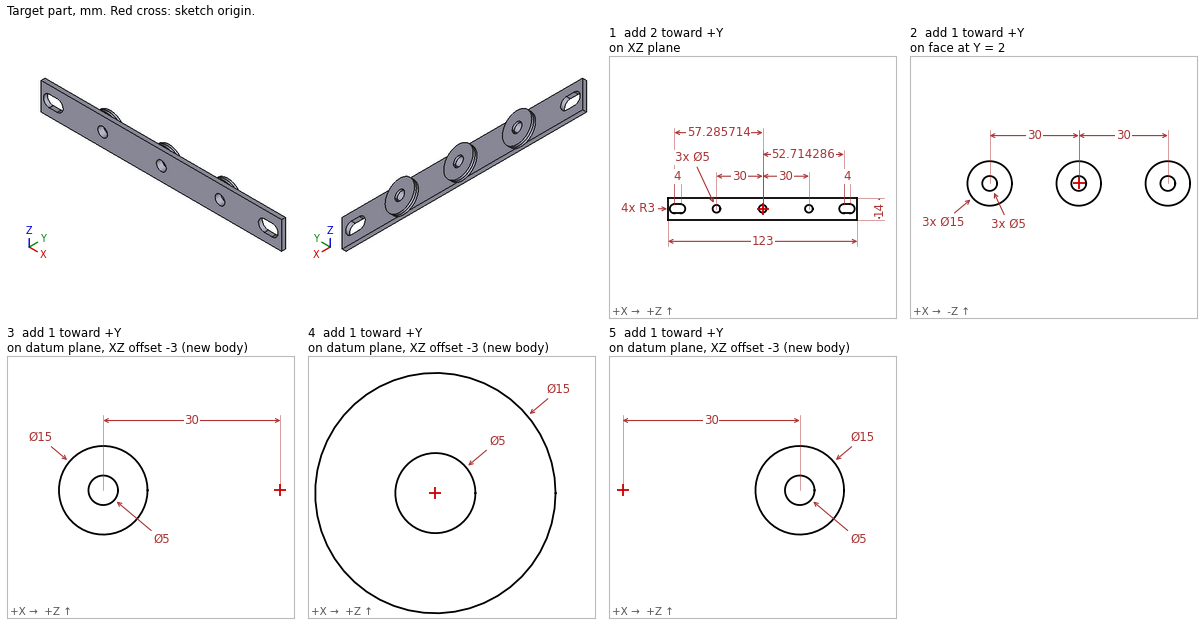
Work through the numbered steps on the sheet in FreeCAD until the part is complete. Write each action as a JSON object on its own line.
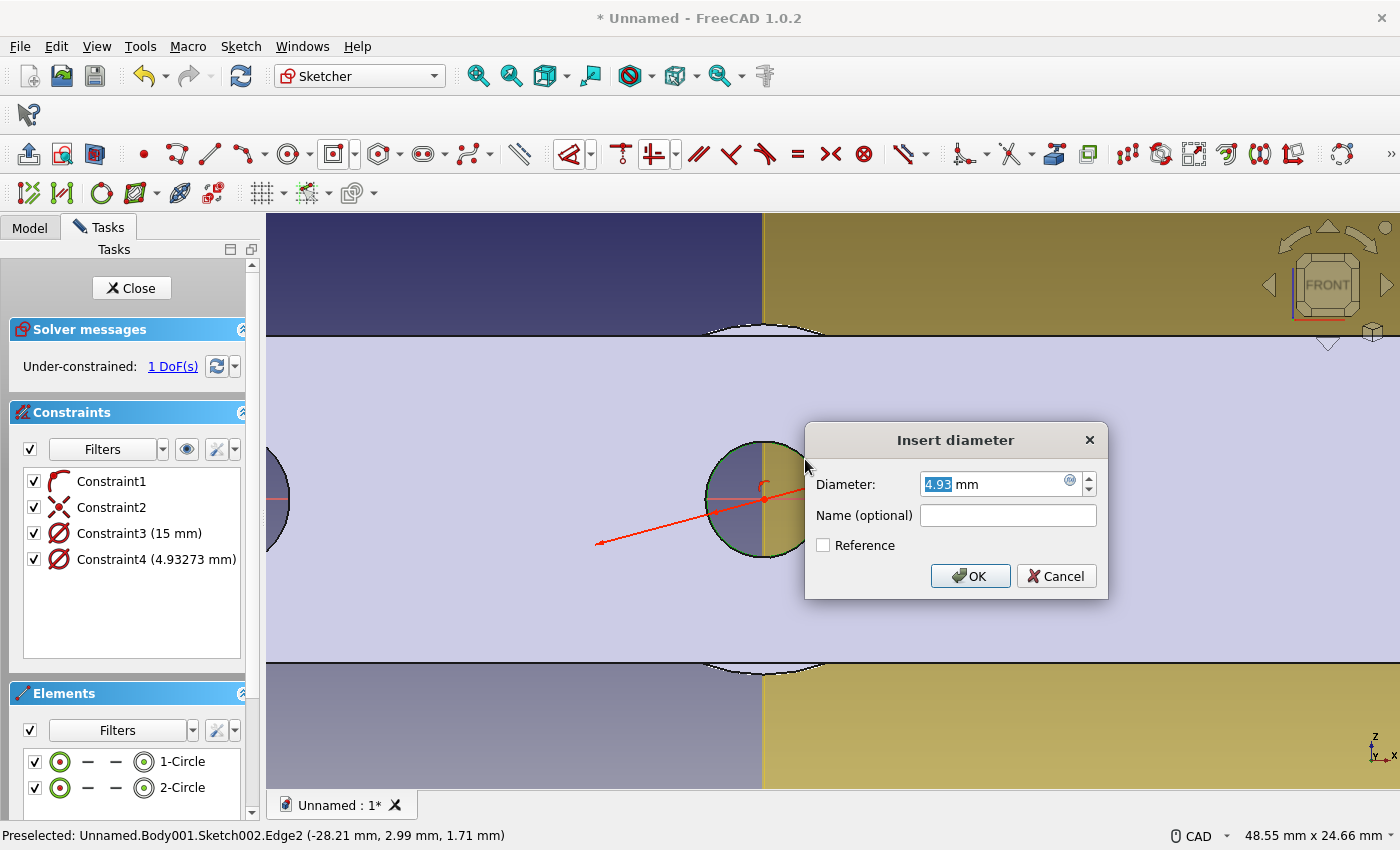
{"action": "type", "text": "5"}
{"action": "key", "text": "Return"}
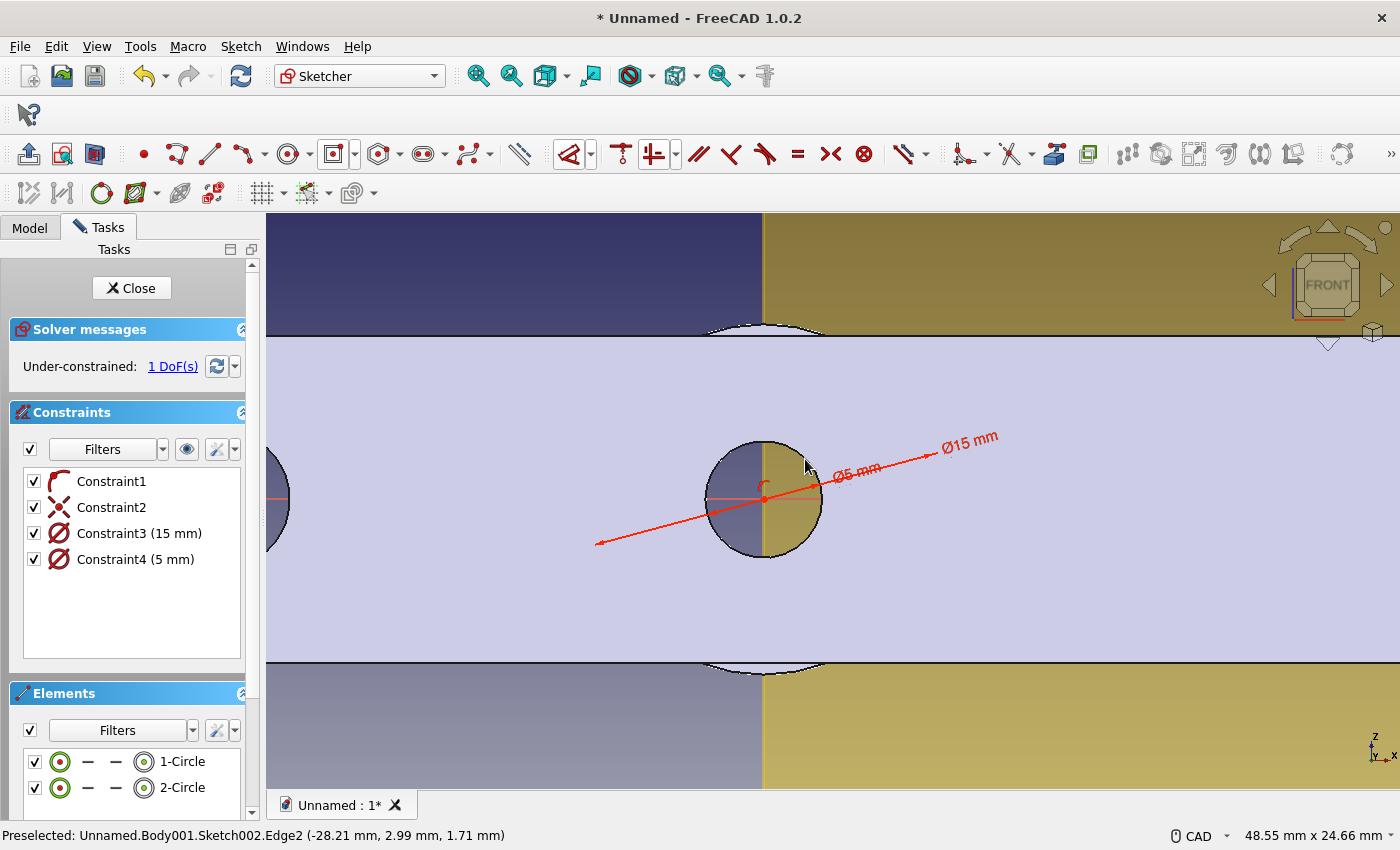
{"action": "left_click", "coordinate": [764, 499]}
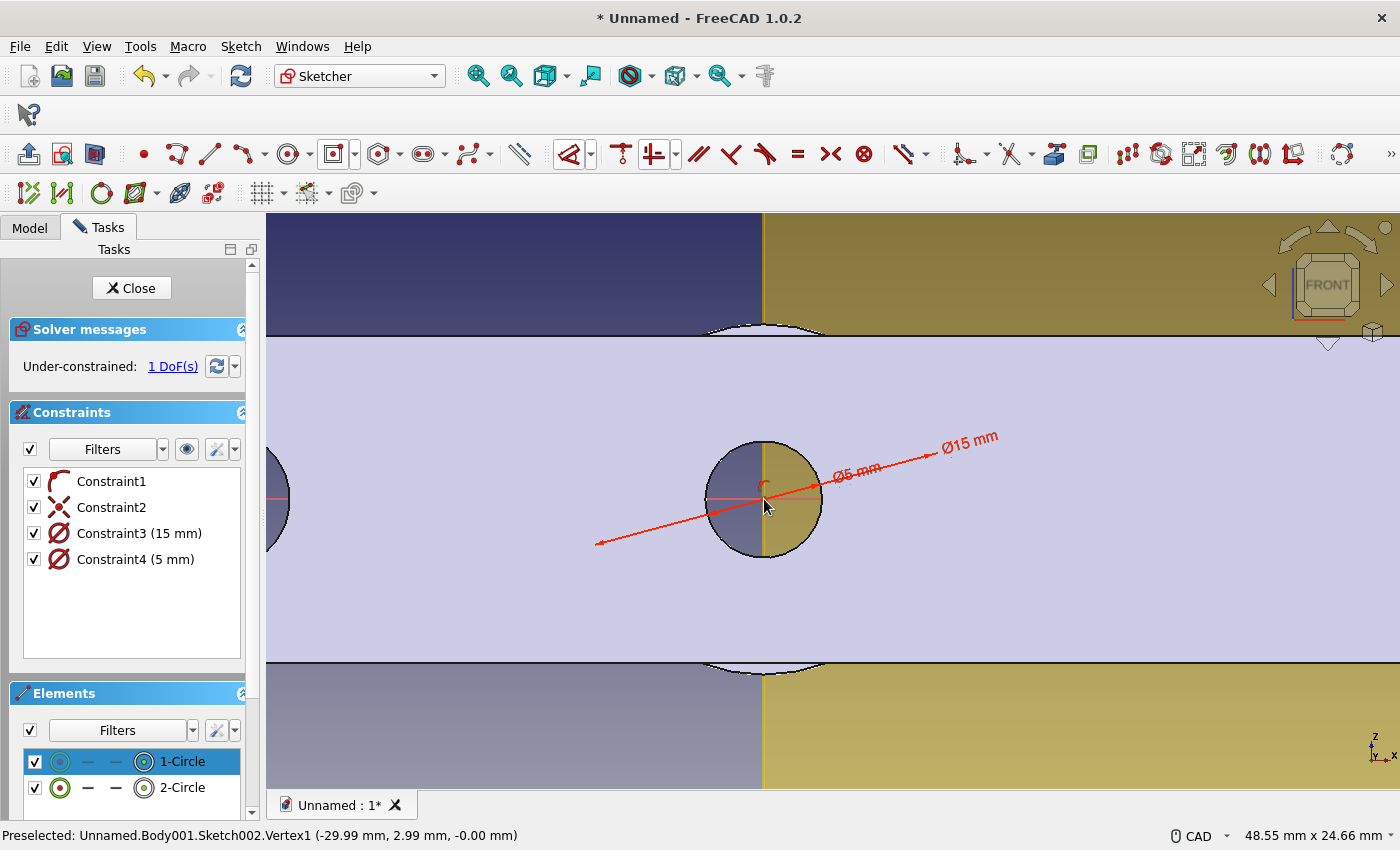
{"action": "left_click", "coordinate": [590, 154]}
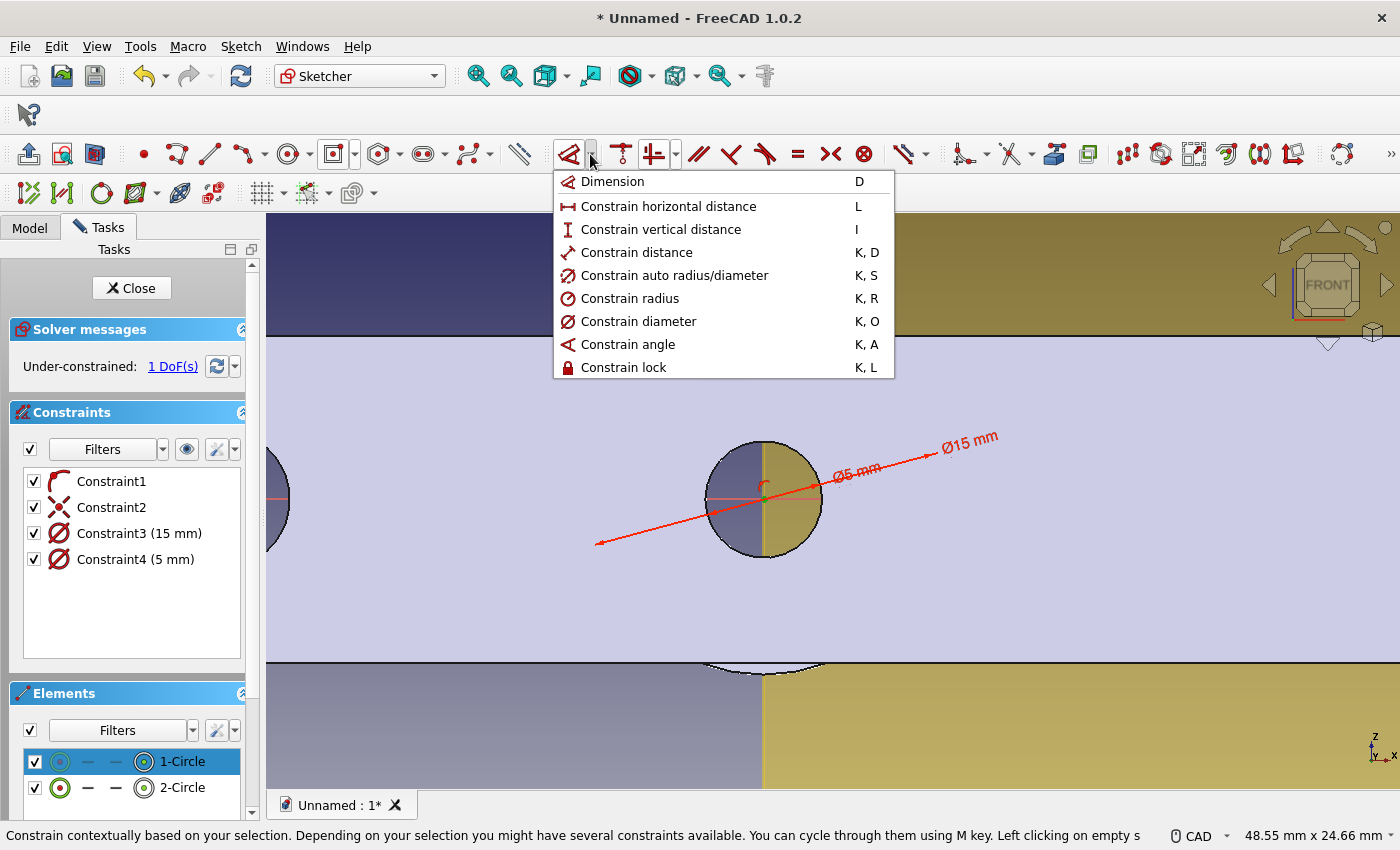
{"action": "left_click", "coordinate": [724, 206]}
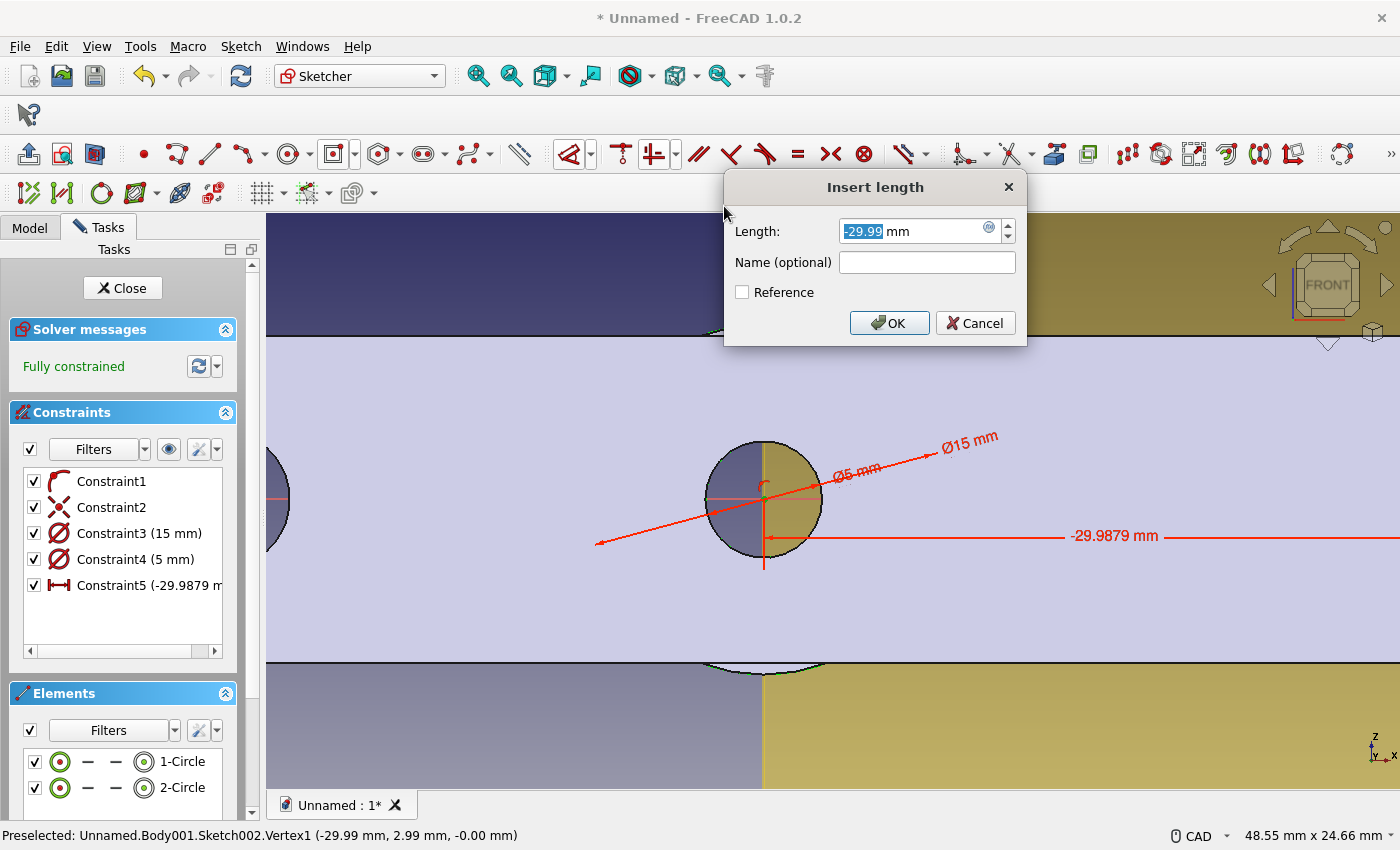
{"action": "type", "text": "-30"}
{"action": "key", "text": "Return"}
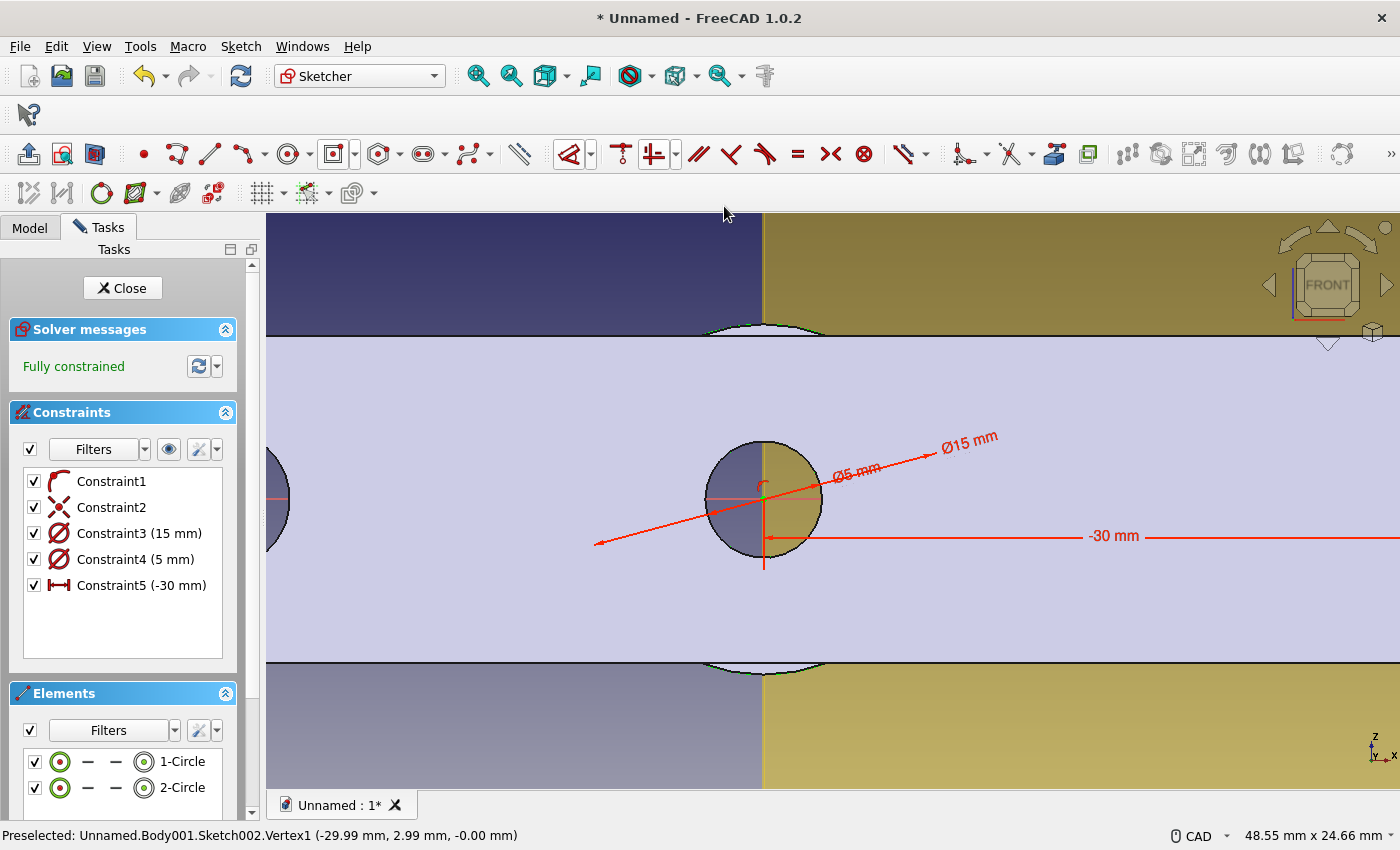
{"action": "left_click", "coordinate": [123, 288]}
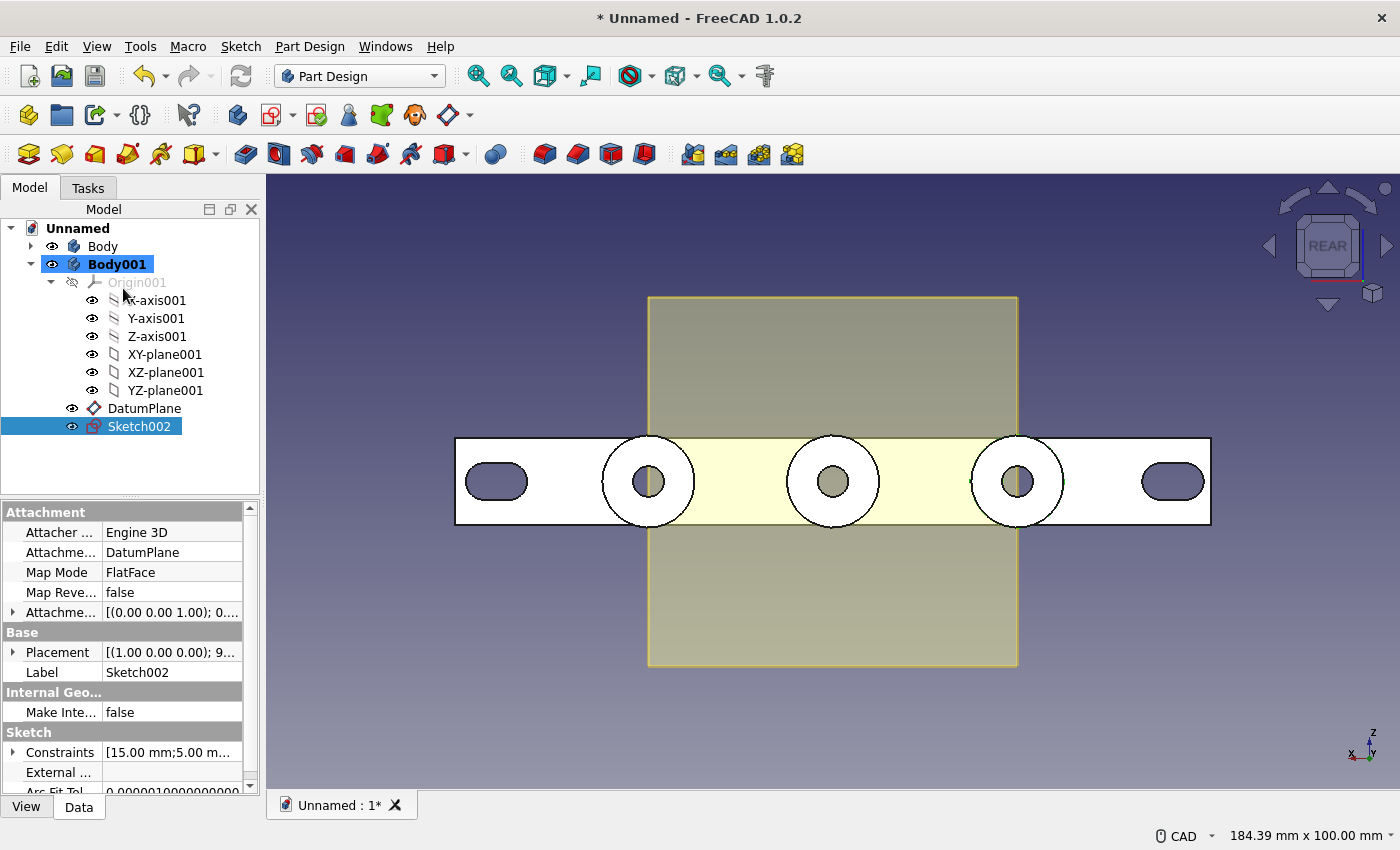
{"action": "left_click", "coordinate": [29, 154]}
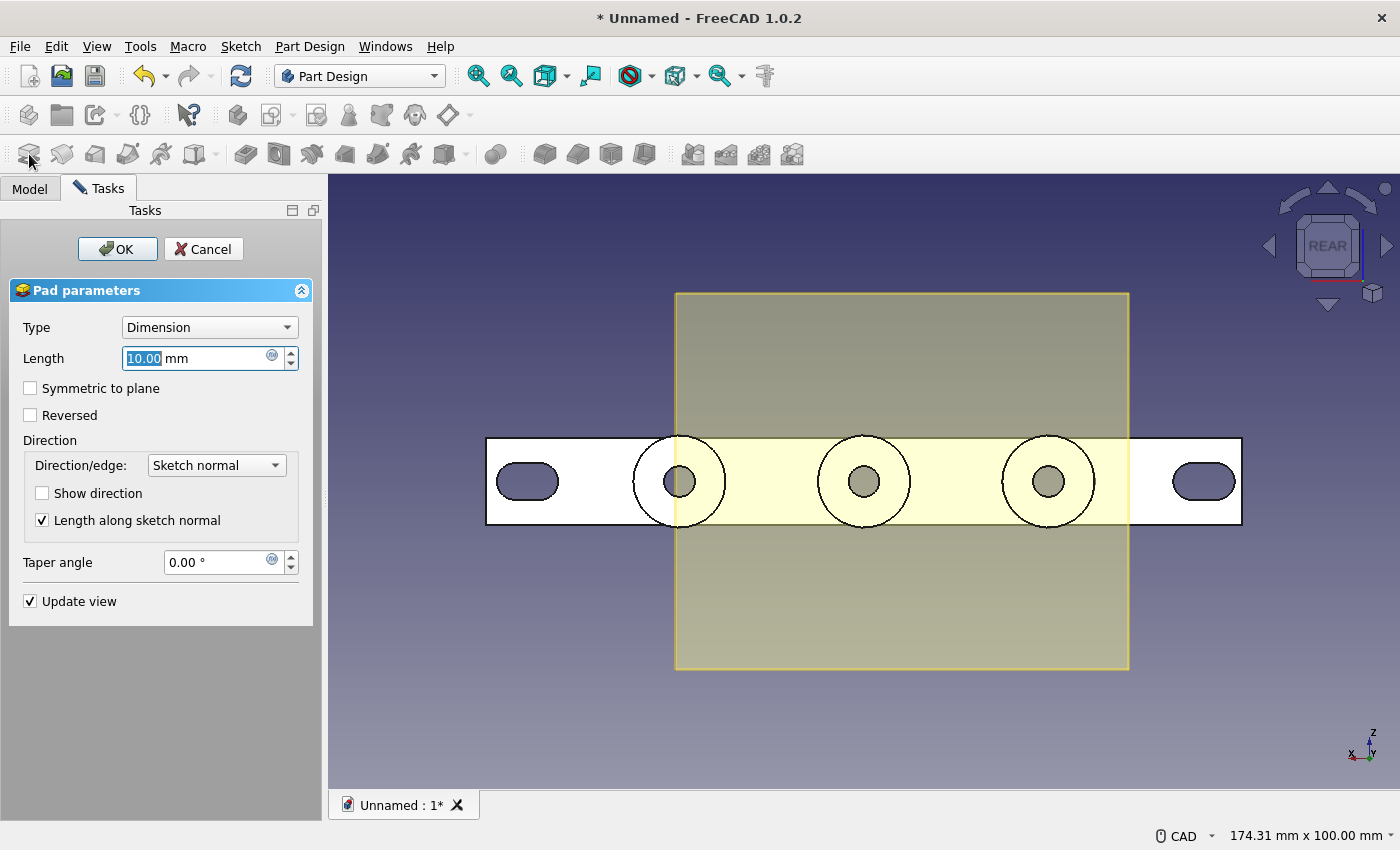
{"action": "type", "text": "1"}
{"action": "key", "text": "Tab"}